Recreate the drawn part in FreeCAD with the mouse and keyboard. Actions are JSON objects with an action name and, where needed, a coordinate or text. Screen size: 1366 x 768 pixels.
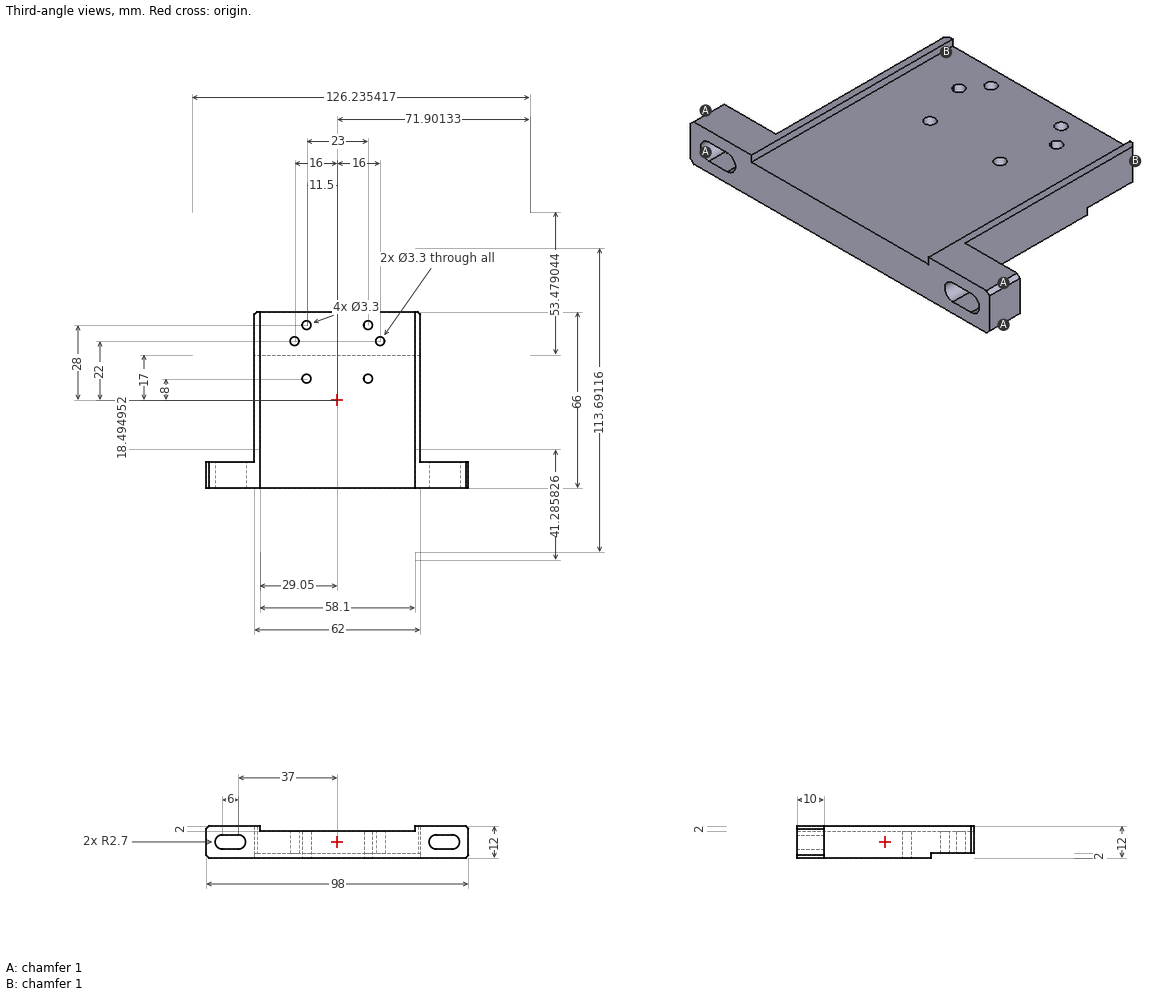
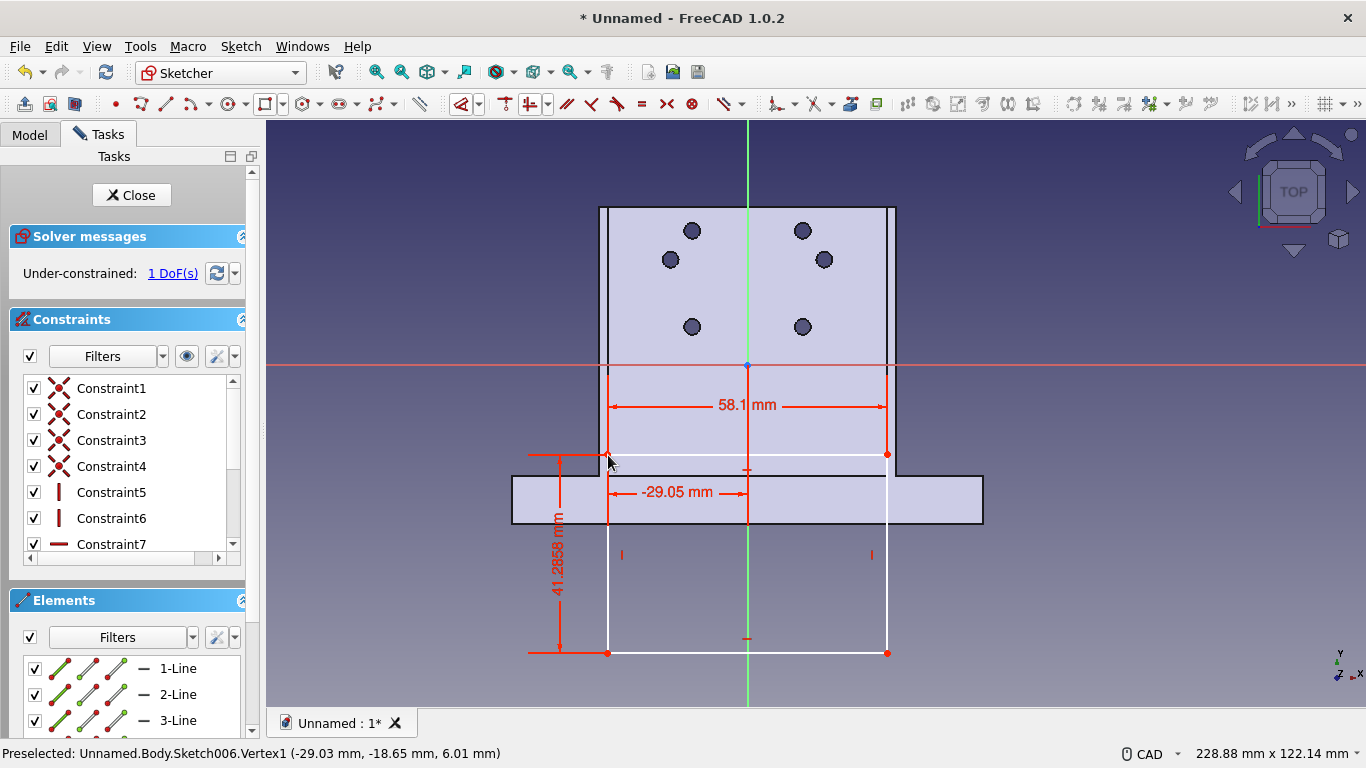
{"action": "left_click", "coordinate": [608, 455]}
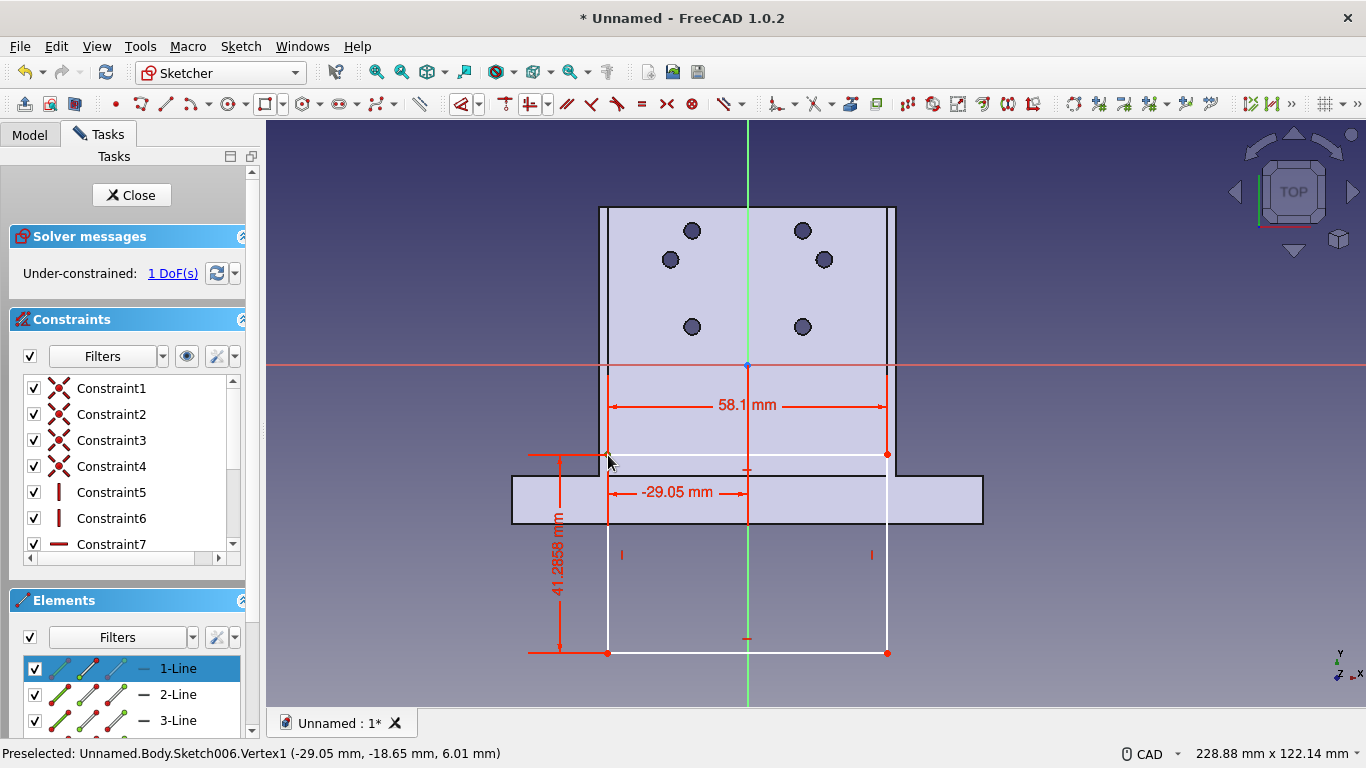
{"action": "key", "text": "i"}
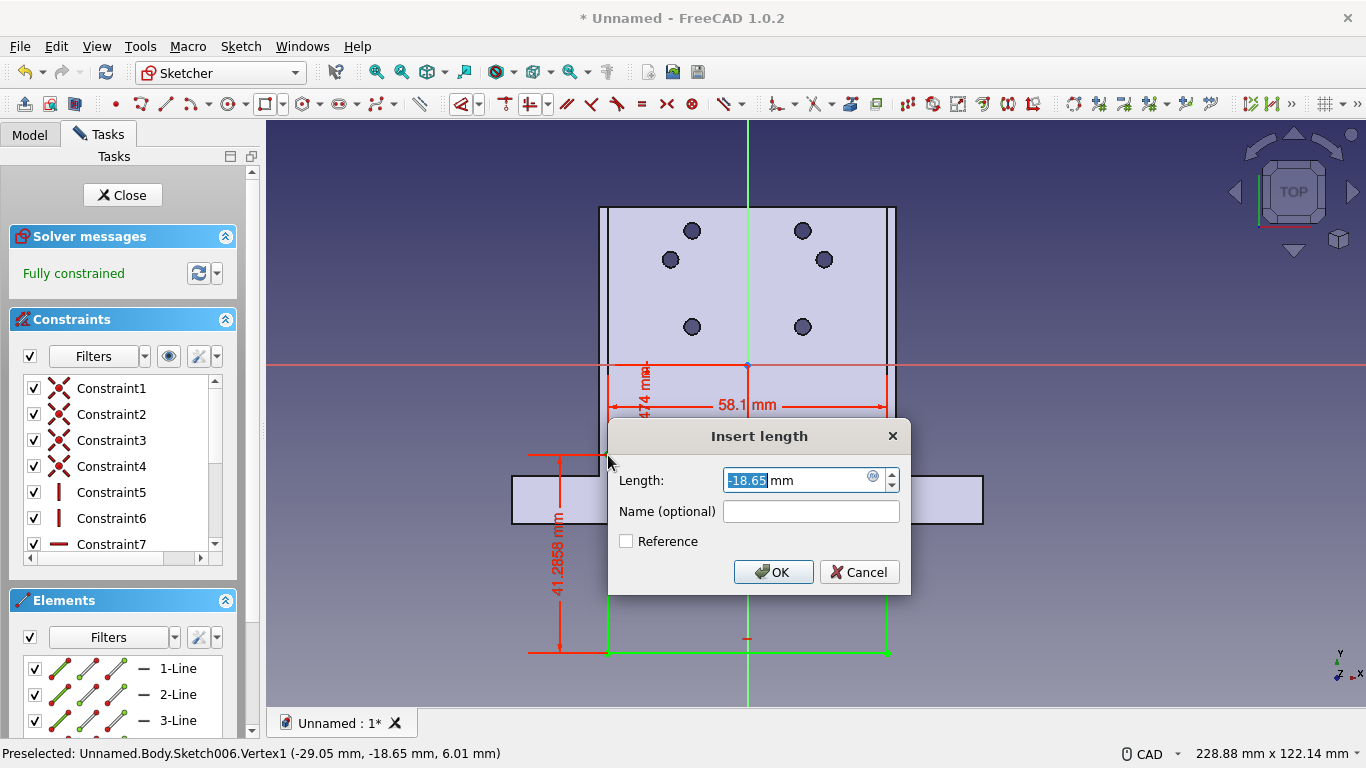
{"action": "type", "text": "-18.494952"}
{"action": "key", "text": "Return"}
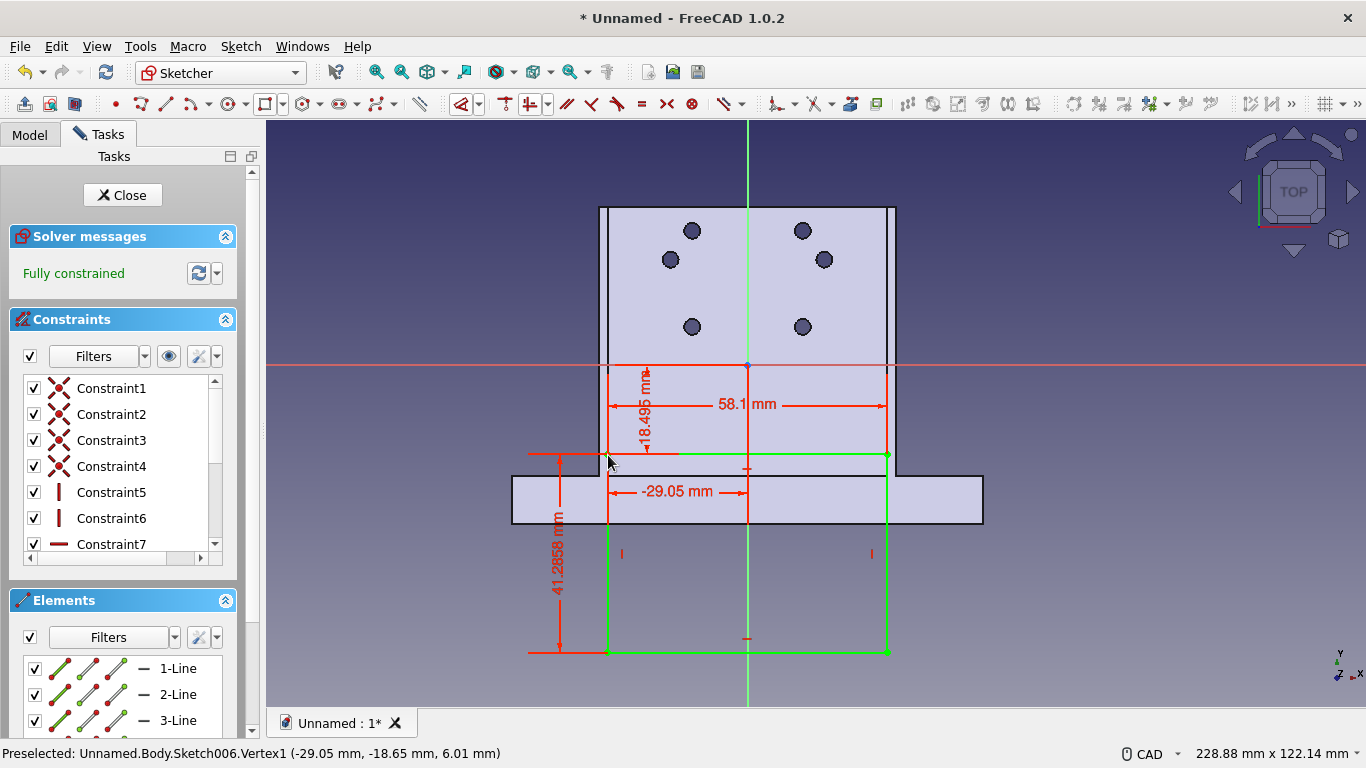
{"action": "left_click", "coordinate": [123, 195]}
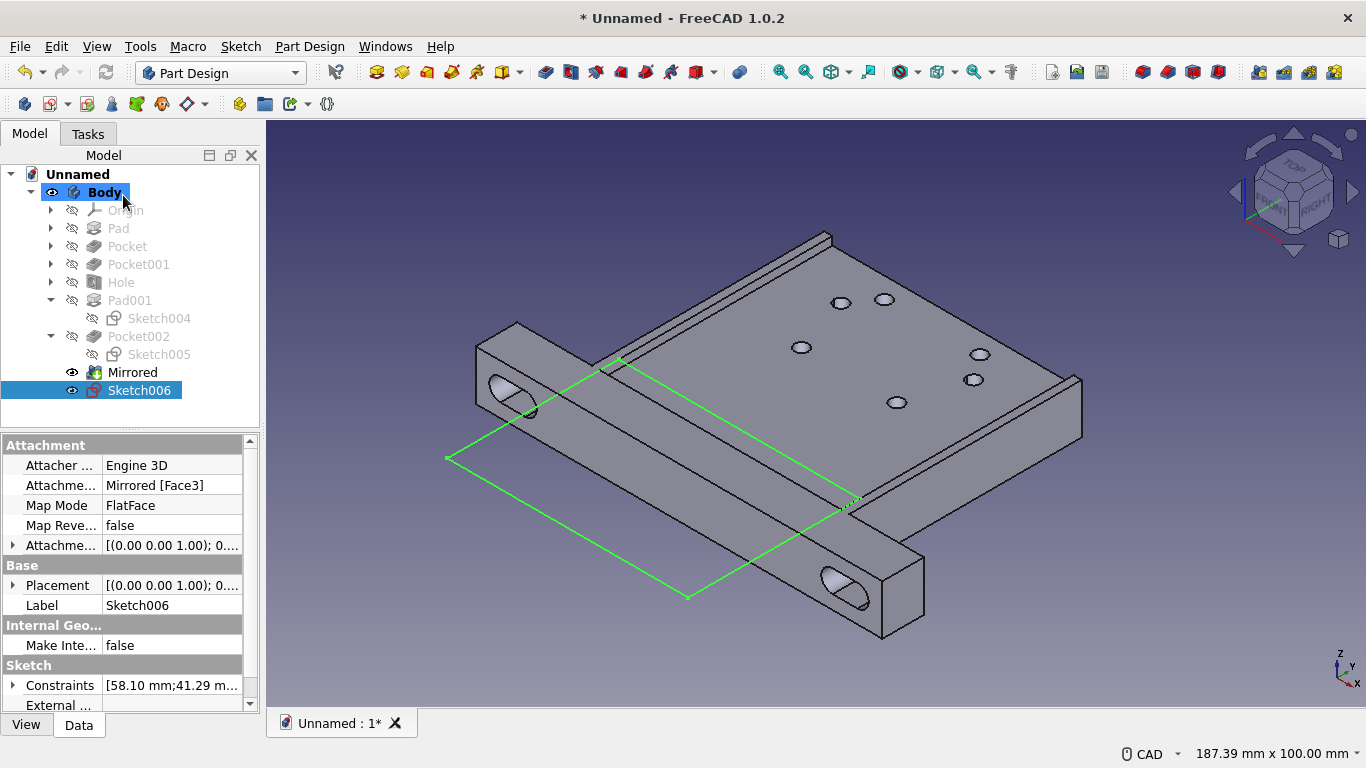
{"action": "left_click", "coordinate": [546, 72]}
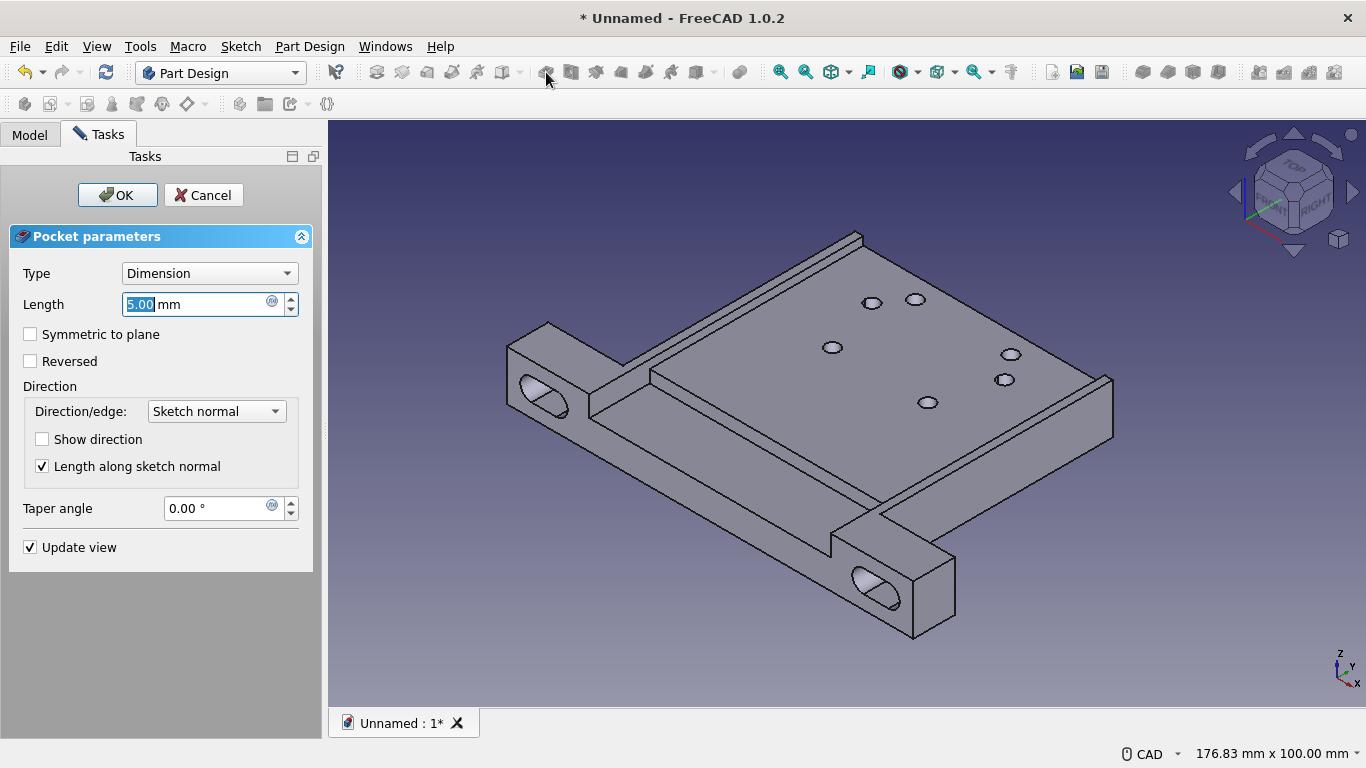
{"action": "type", "text": "2"}
{"action": "key", "text": "Tab"}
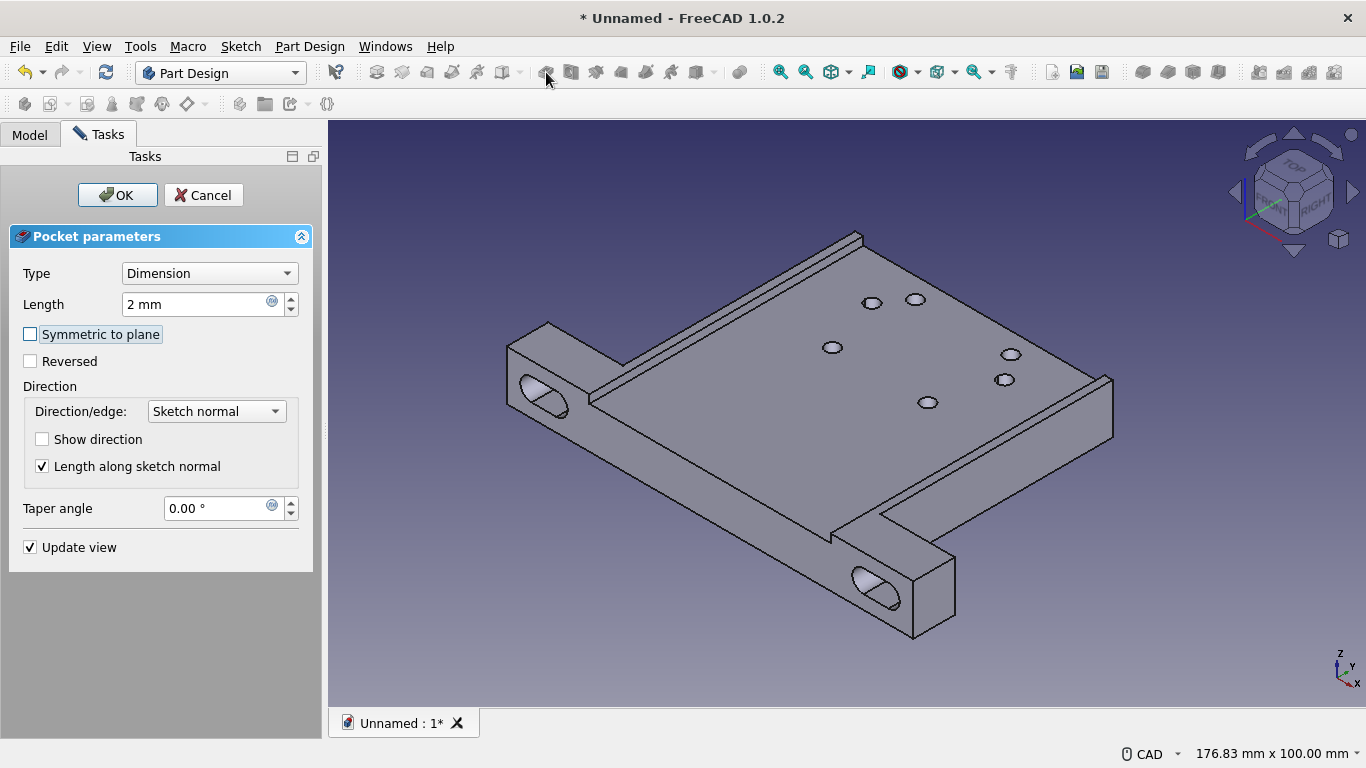
{"action": "left_click", "coordinate": [118, 195]}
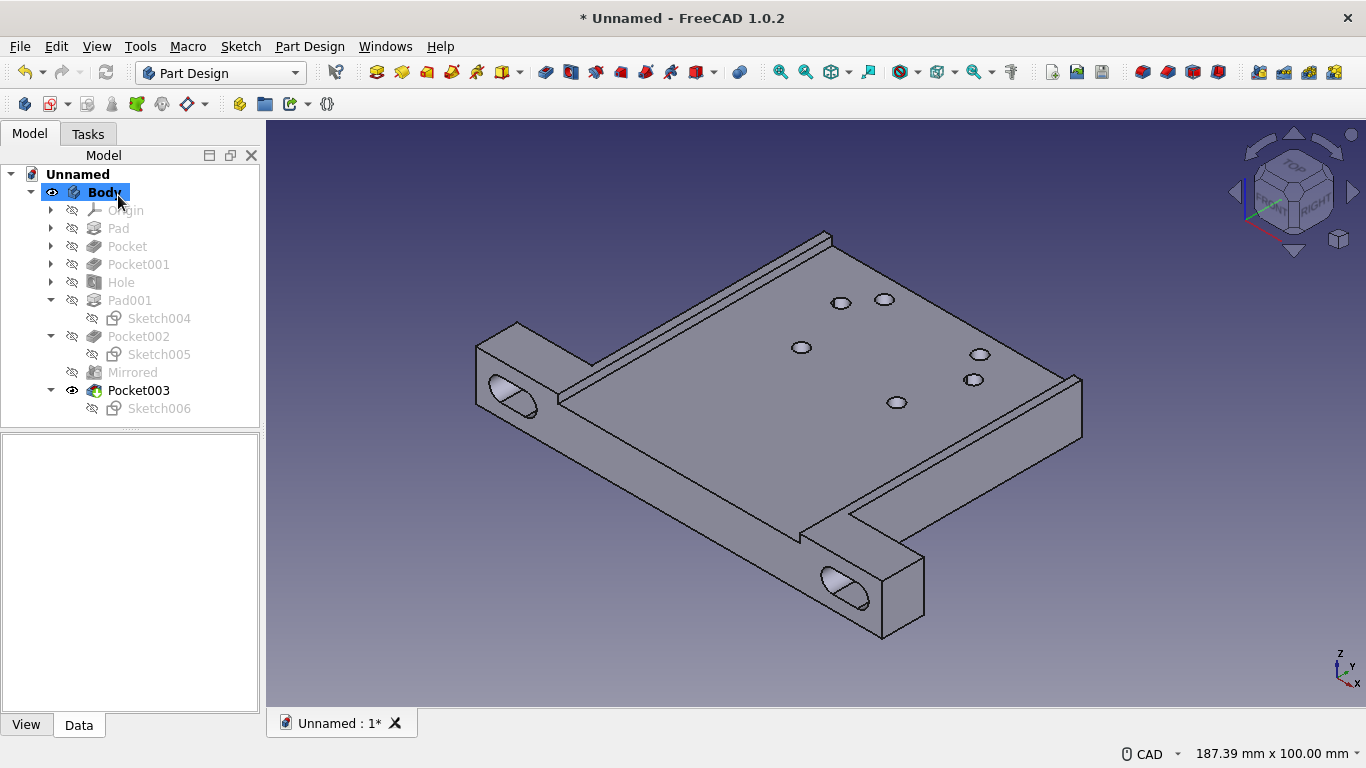
{"action": "key", "text": "5"}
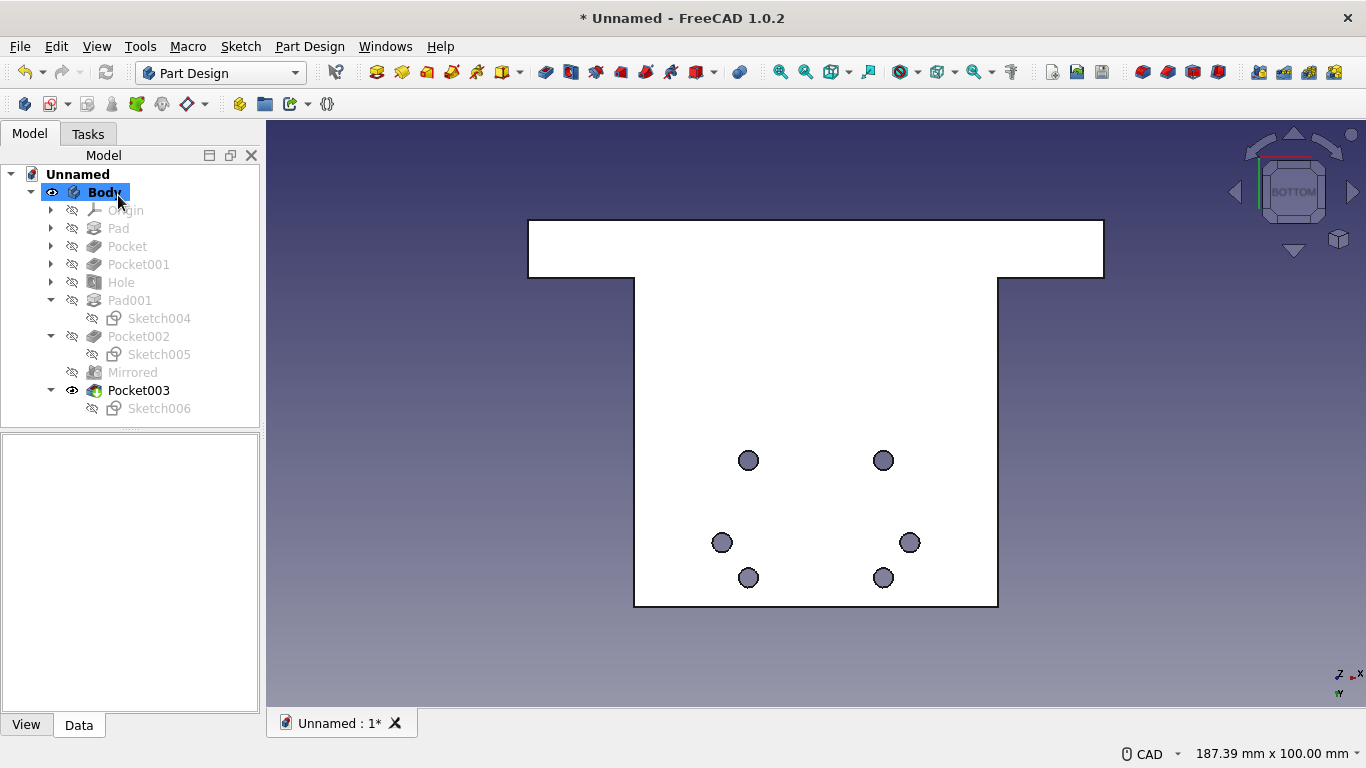
{"action": "left_click", "coordinate": [816, 357]}